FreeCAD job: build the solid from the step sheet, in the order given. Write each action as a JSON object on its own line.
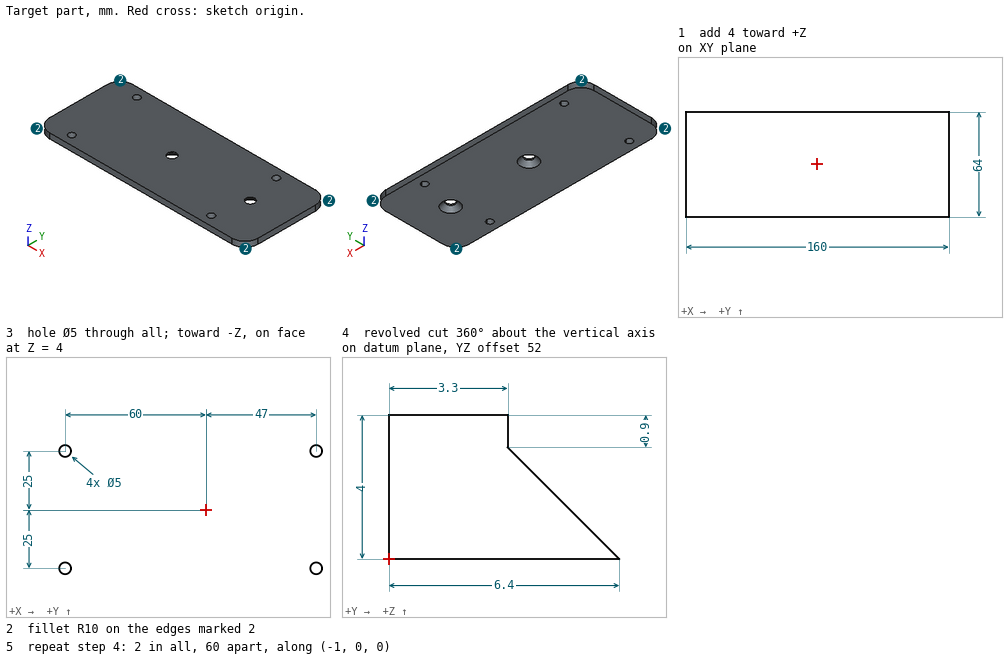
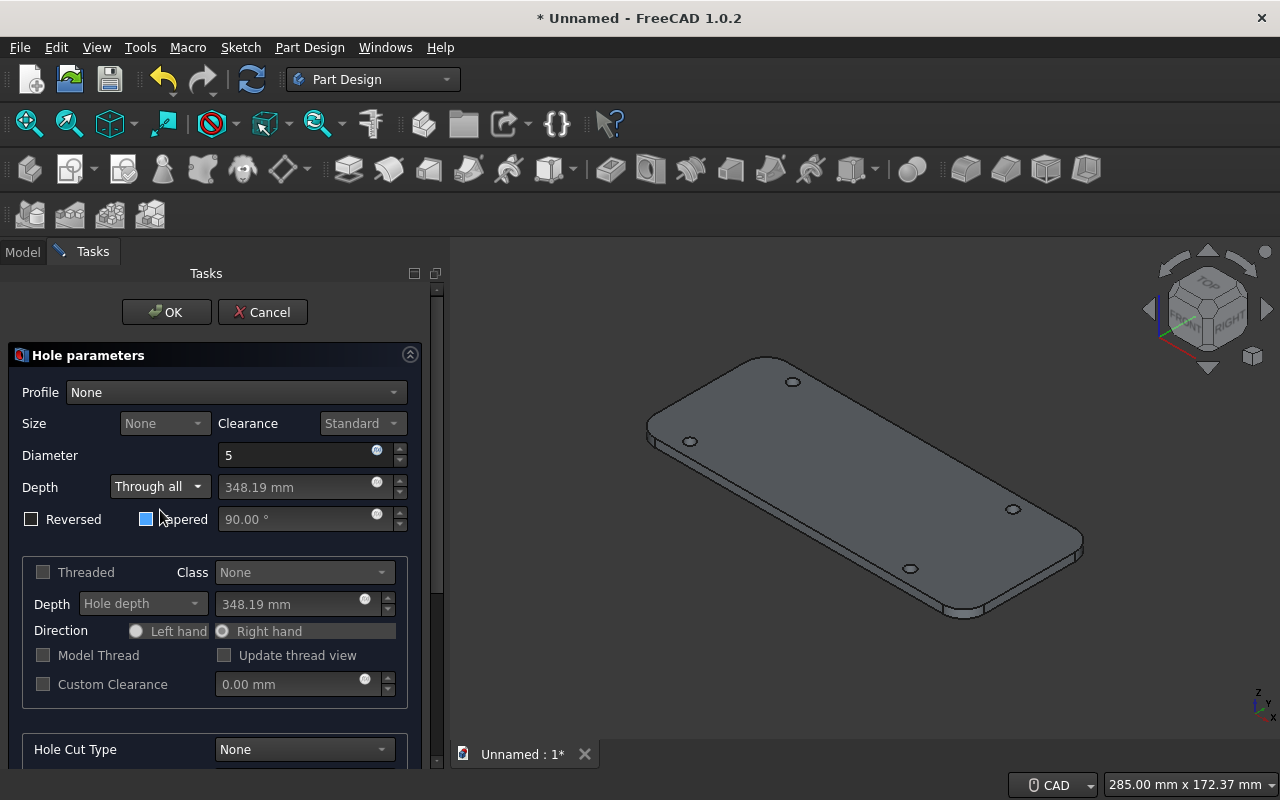
{"action": "left_click", "coordinate": [167, 312]}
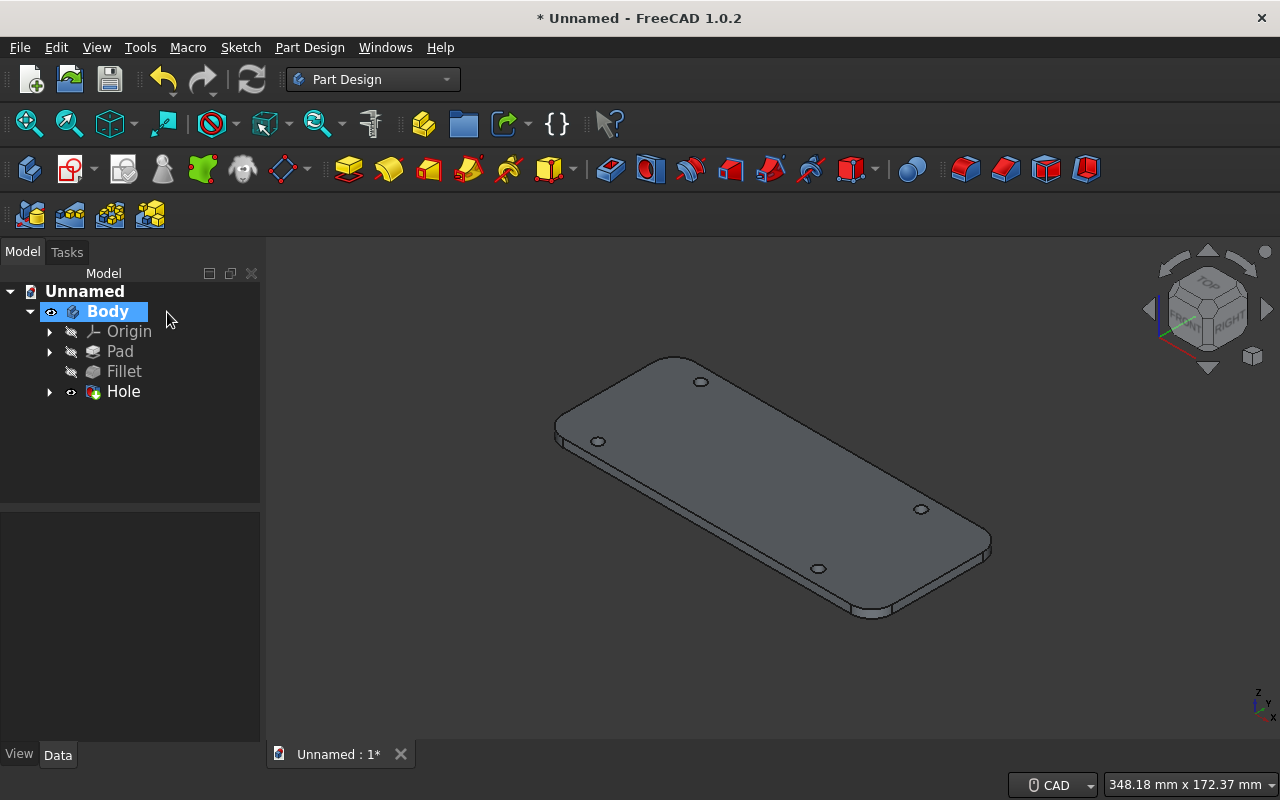
{"action": "left_click", "coordinate": [50, 332]}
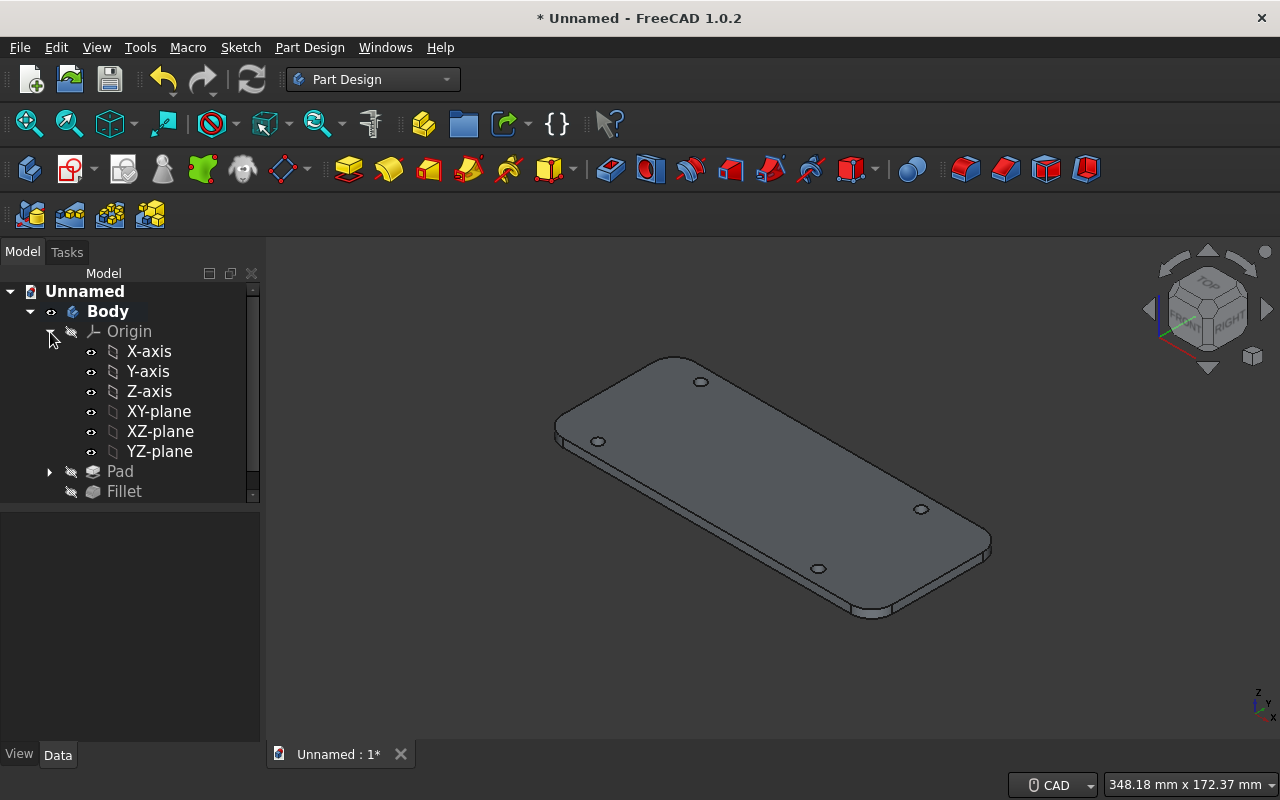
{"action": "left_click", "coordinate": [136, 452]}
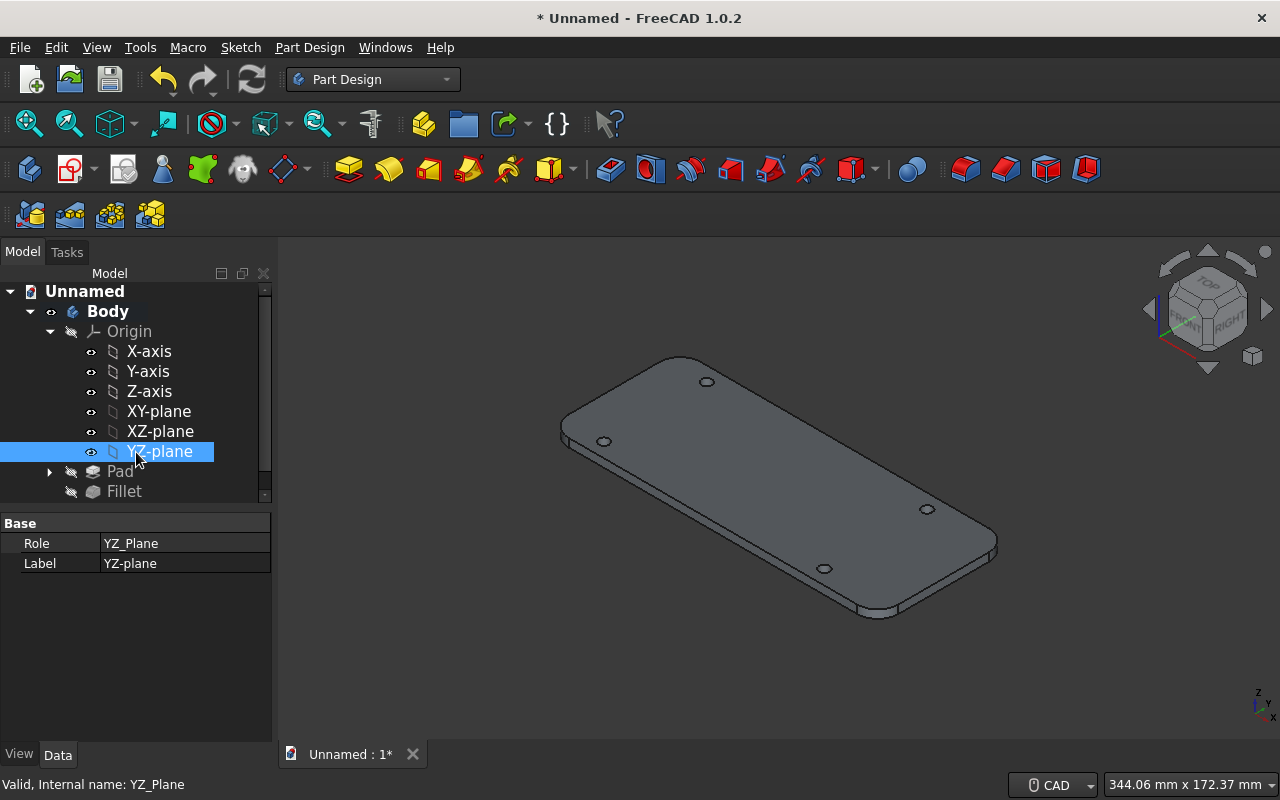
{"action": "left_click", "coordinate": [284, 170]}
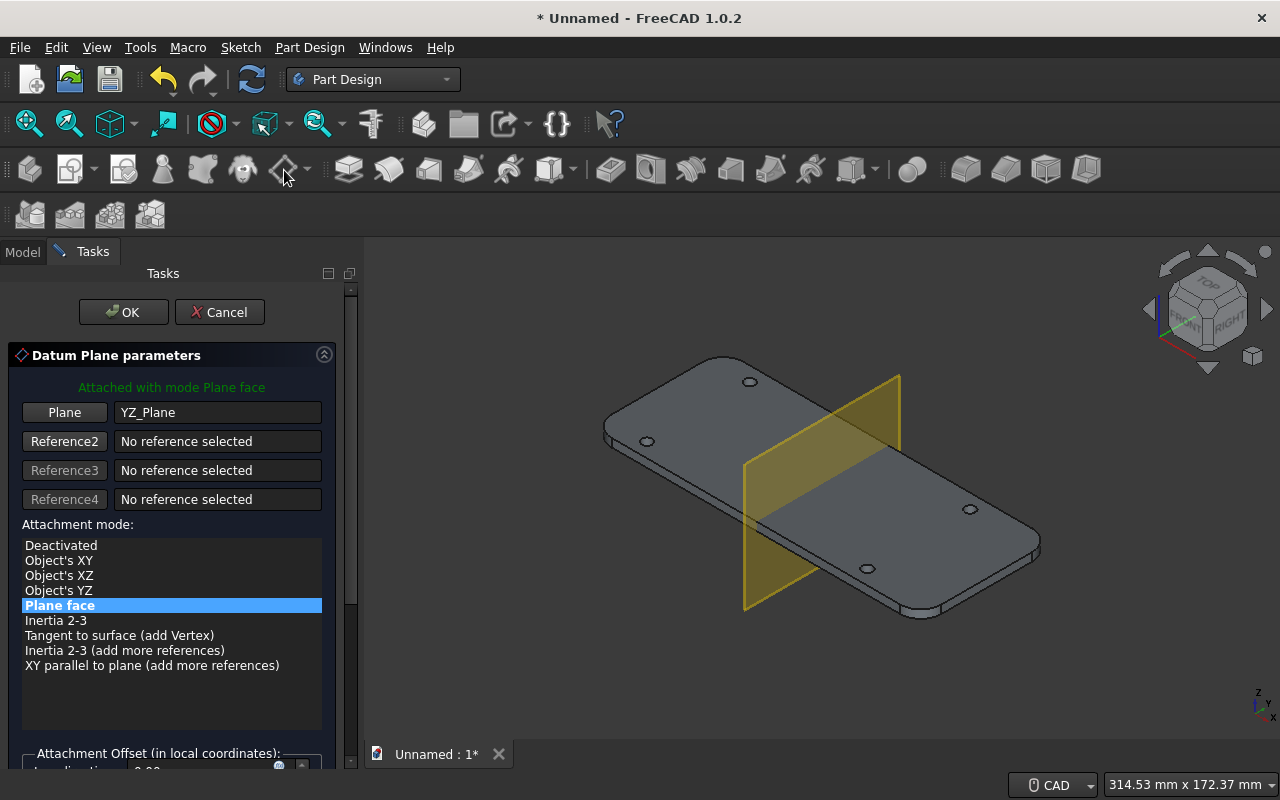
{"action": "scroll", "coordinate": [351, 526], "scroll_direction": "down", "scroll_amount": 3}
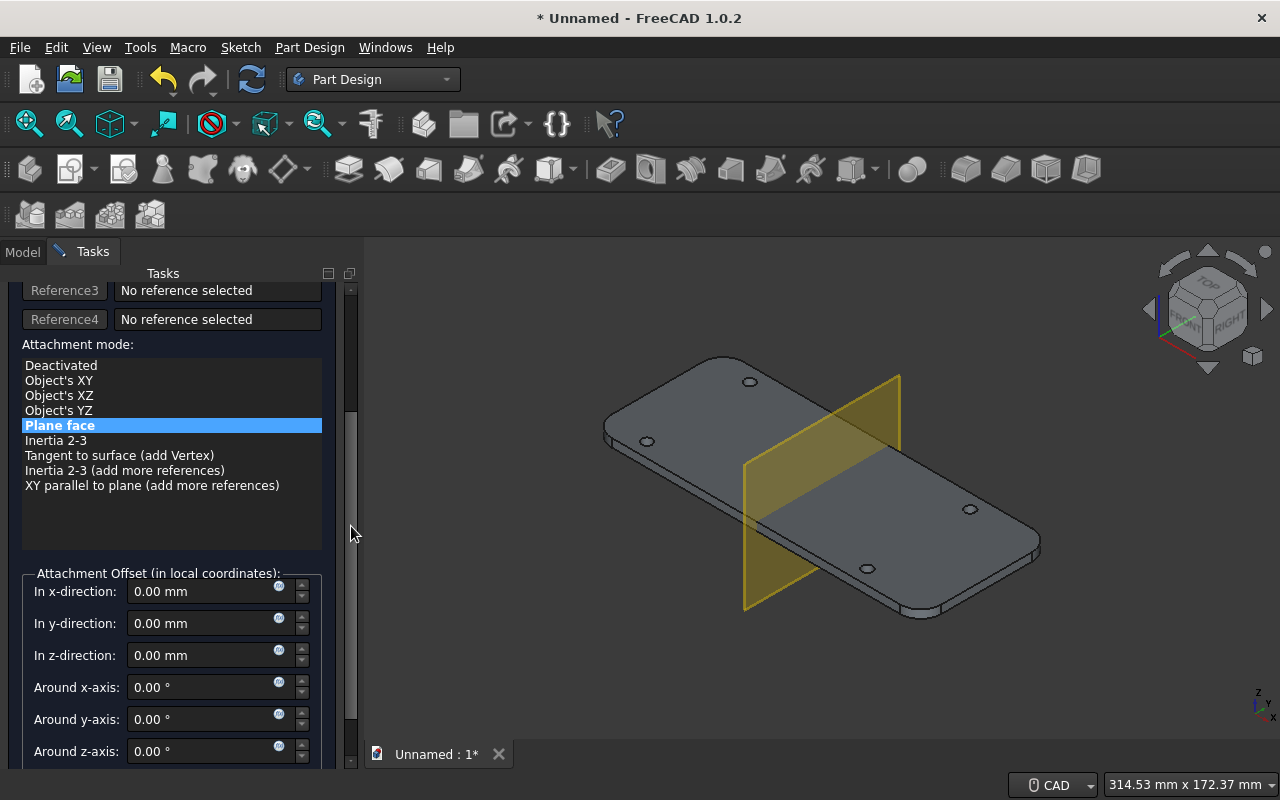
{"action": "triple_click", "coordinate": [210, 655]}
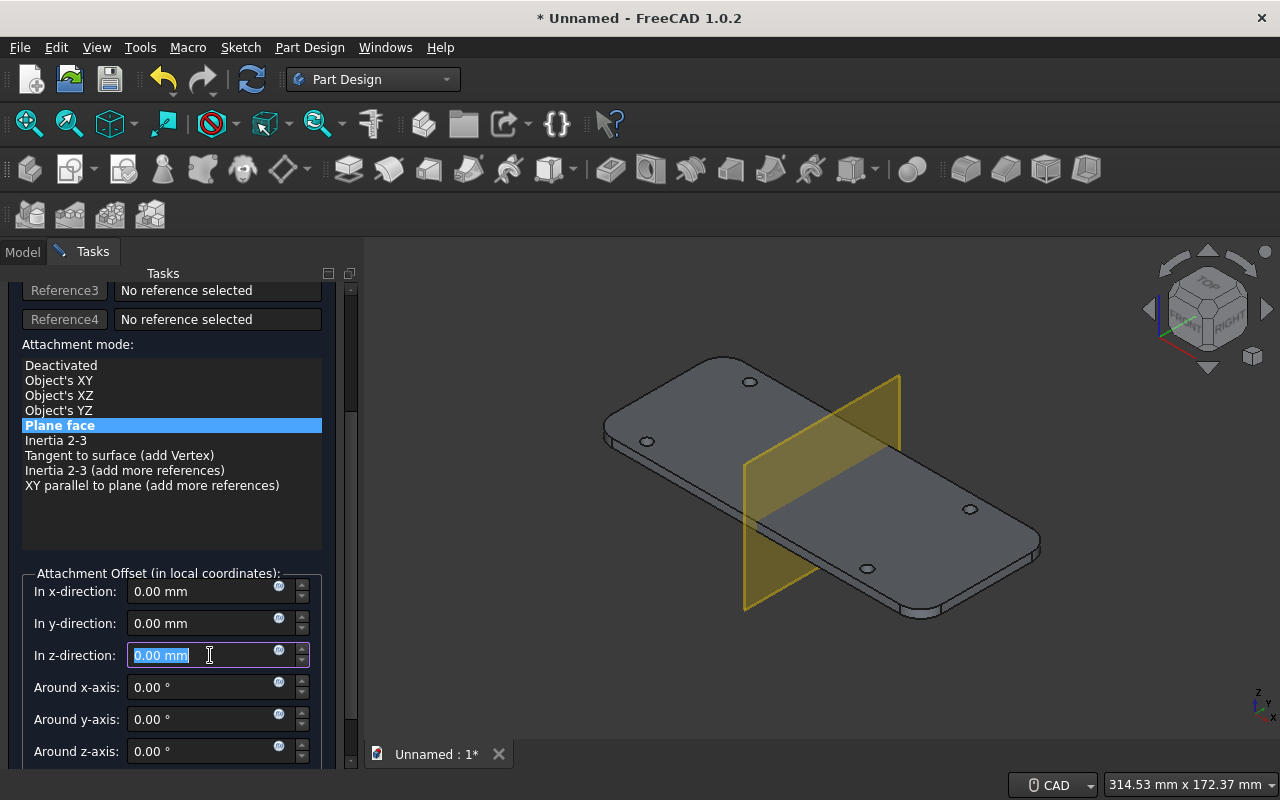
{"action": "type", "text": "52"}
{"action": "key", "text": "Tab"}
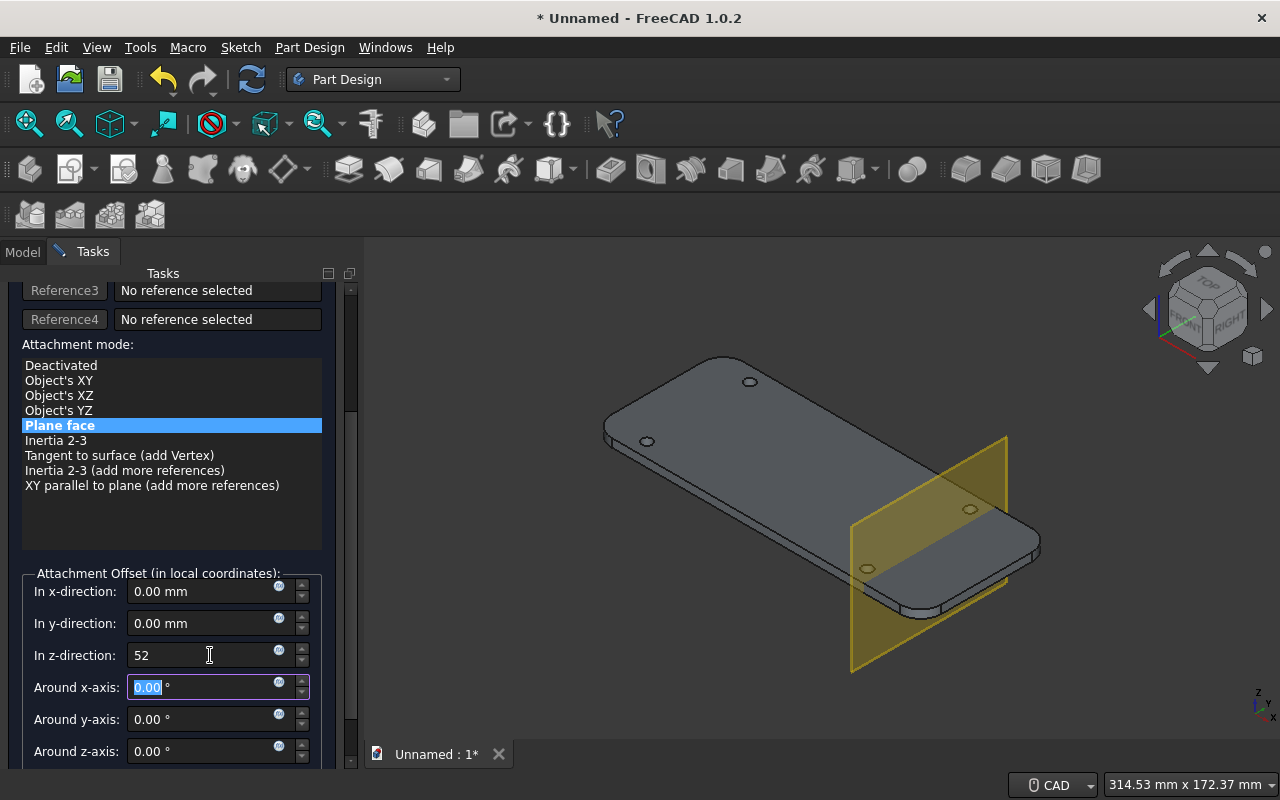
{"action": "scroll", "coordinate": [351, 526], "scroll_direction": "up", "scroll_amount": 4}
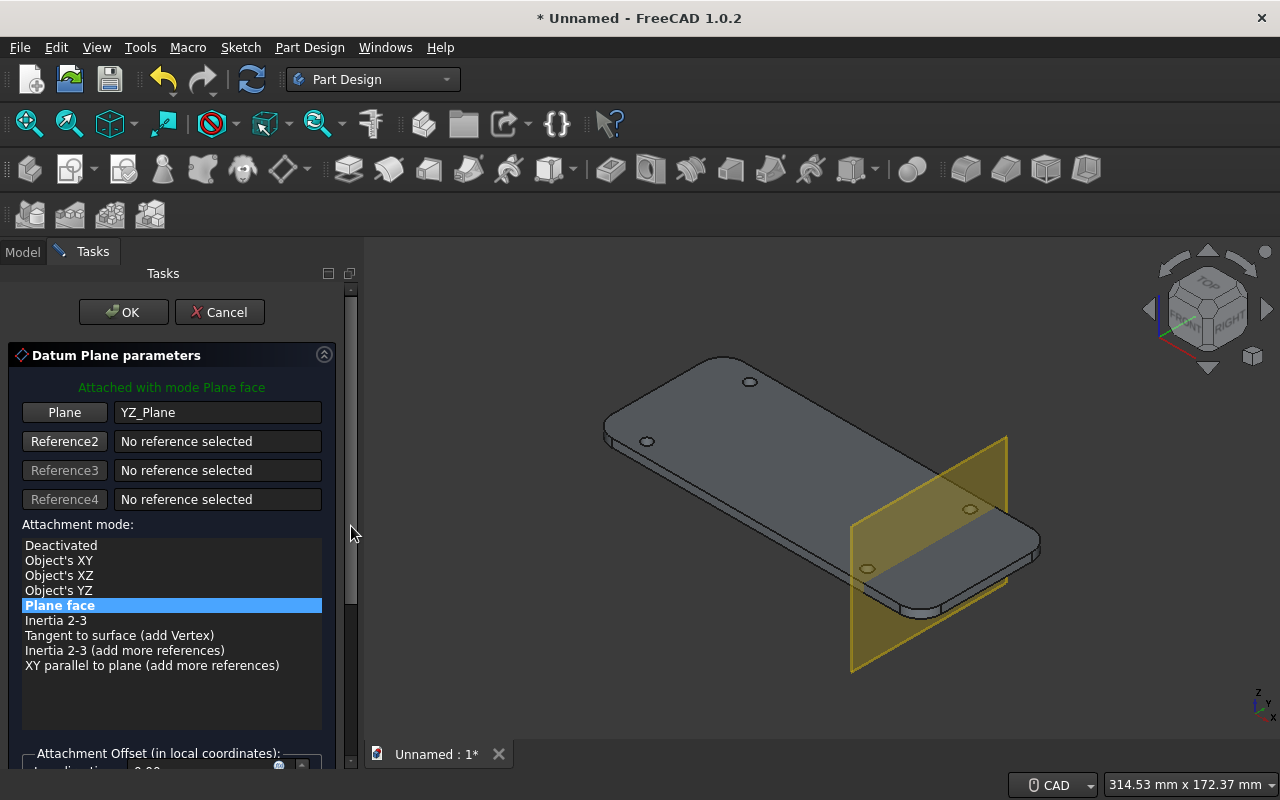
{"action": "left_click", "coordinate": [124, 312]}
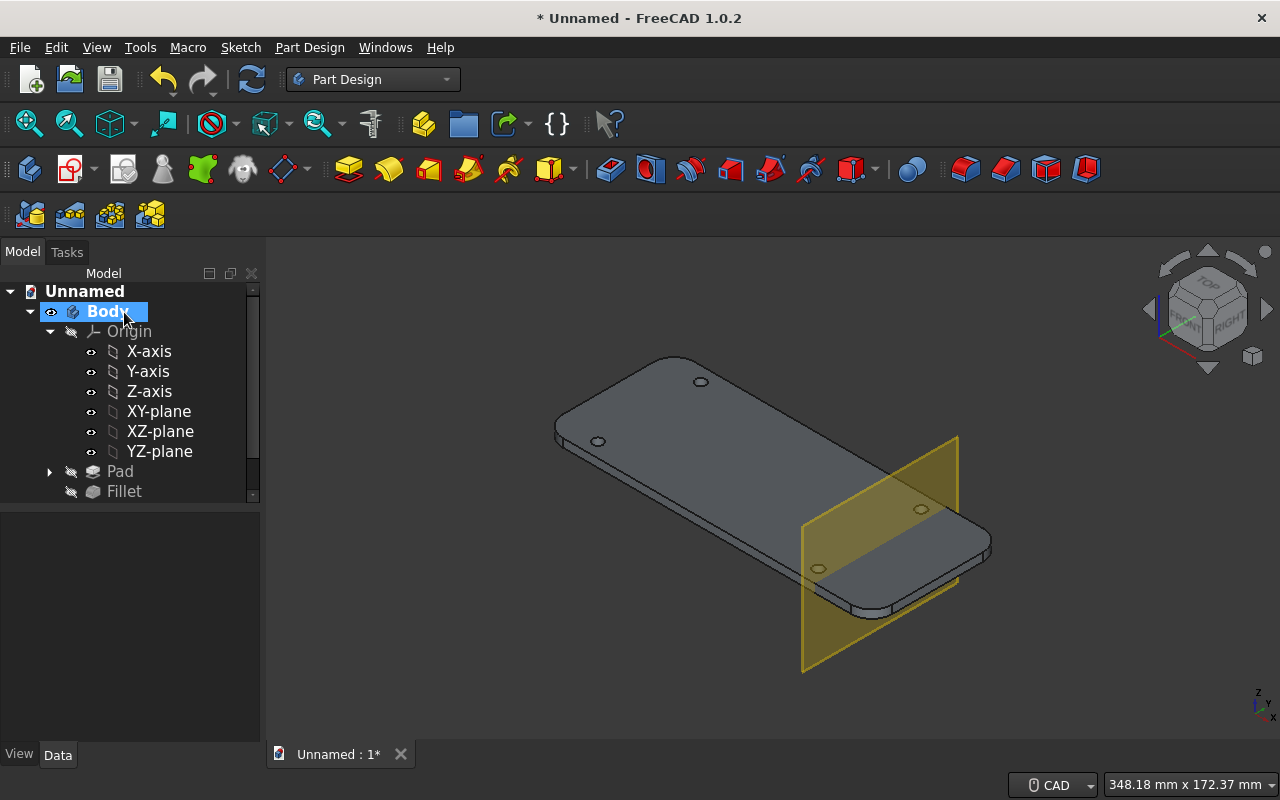
{"action": "scroll", "coordinate": [100, 387], "scroll_direction": "down", "scroll_amount": 3}